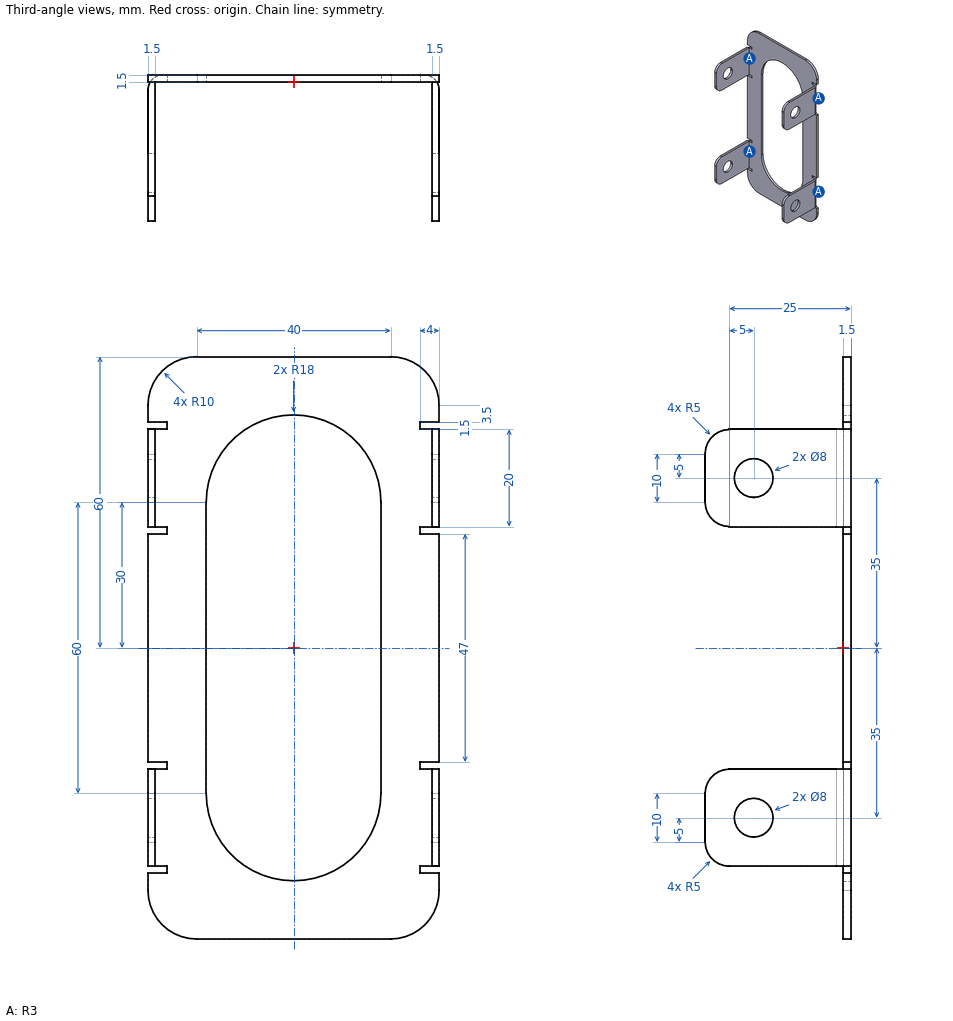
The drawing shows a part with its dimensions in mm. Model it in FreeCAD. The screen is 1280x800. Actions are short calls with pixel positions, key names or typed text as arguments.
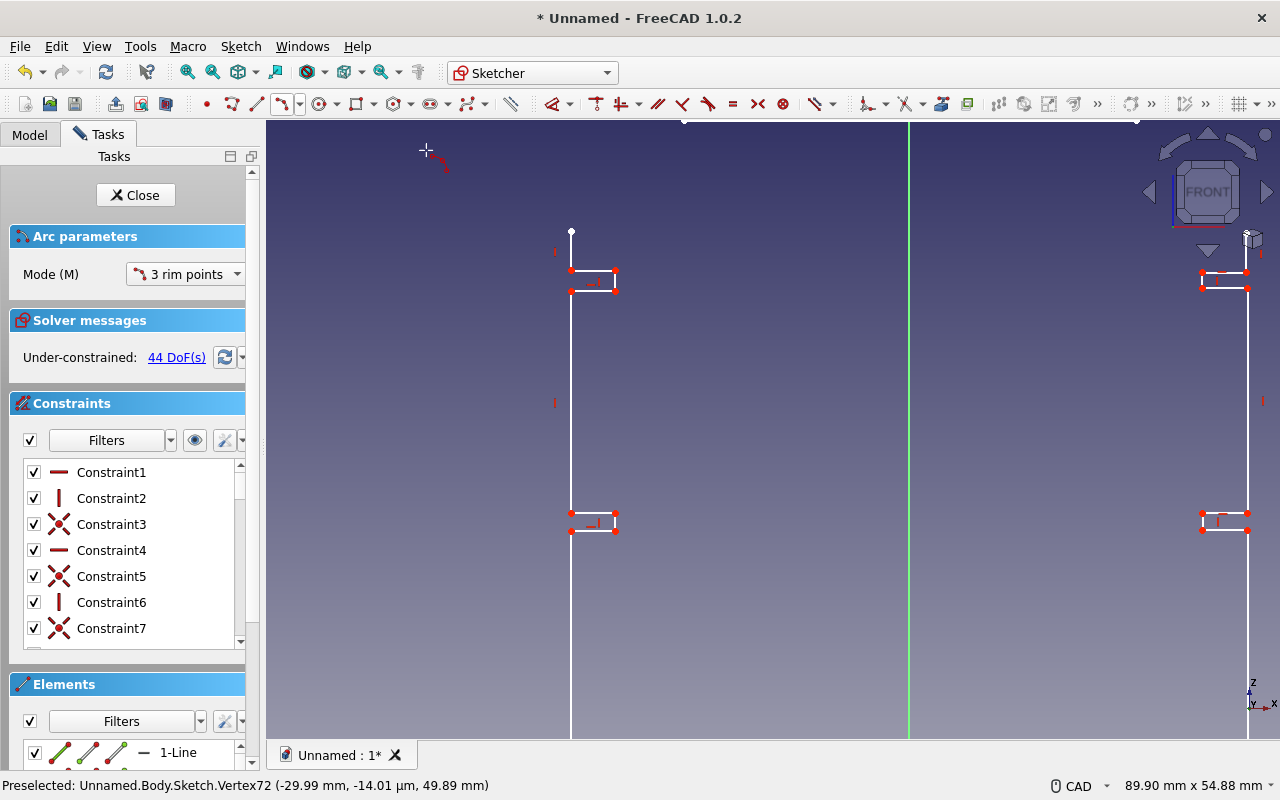
scroll(616, 272, down, 6)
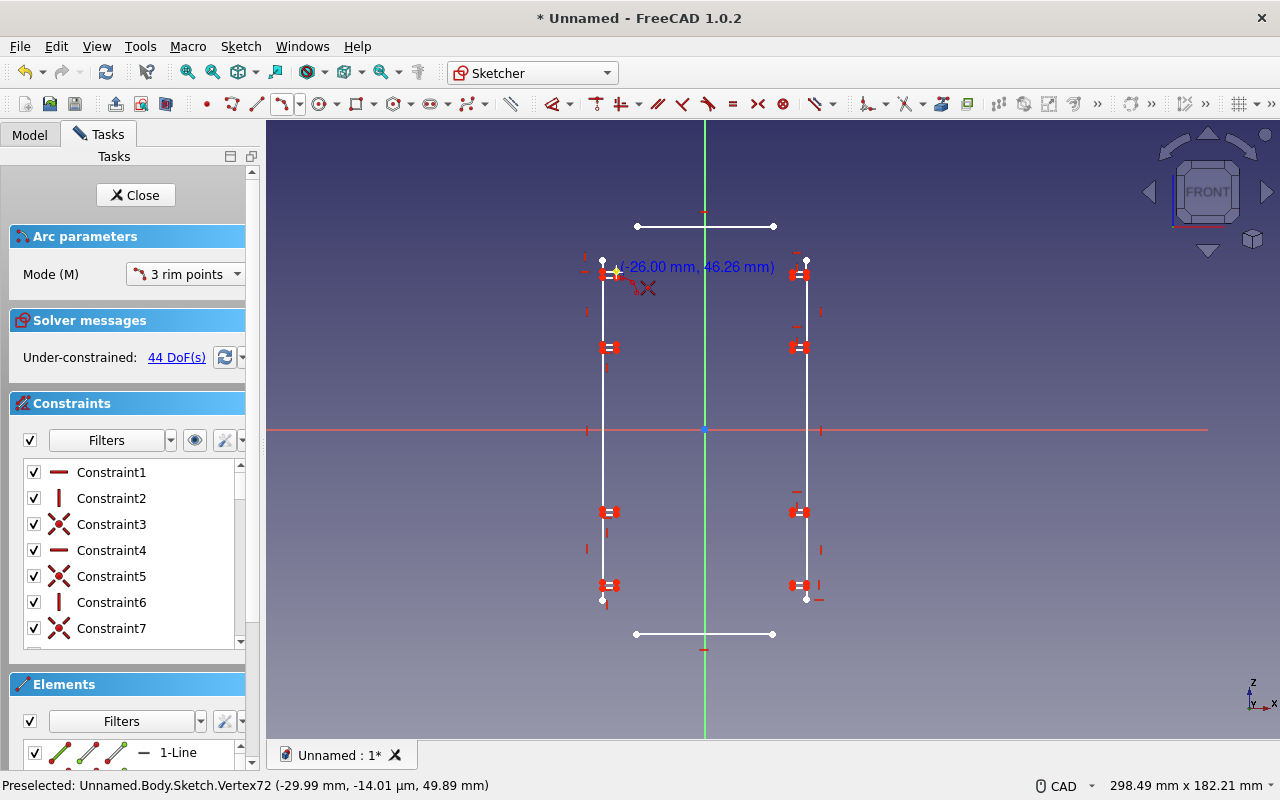
click(773, 227)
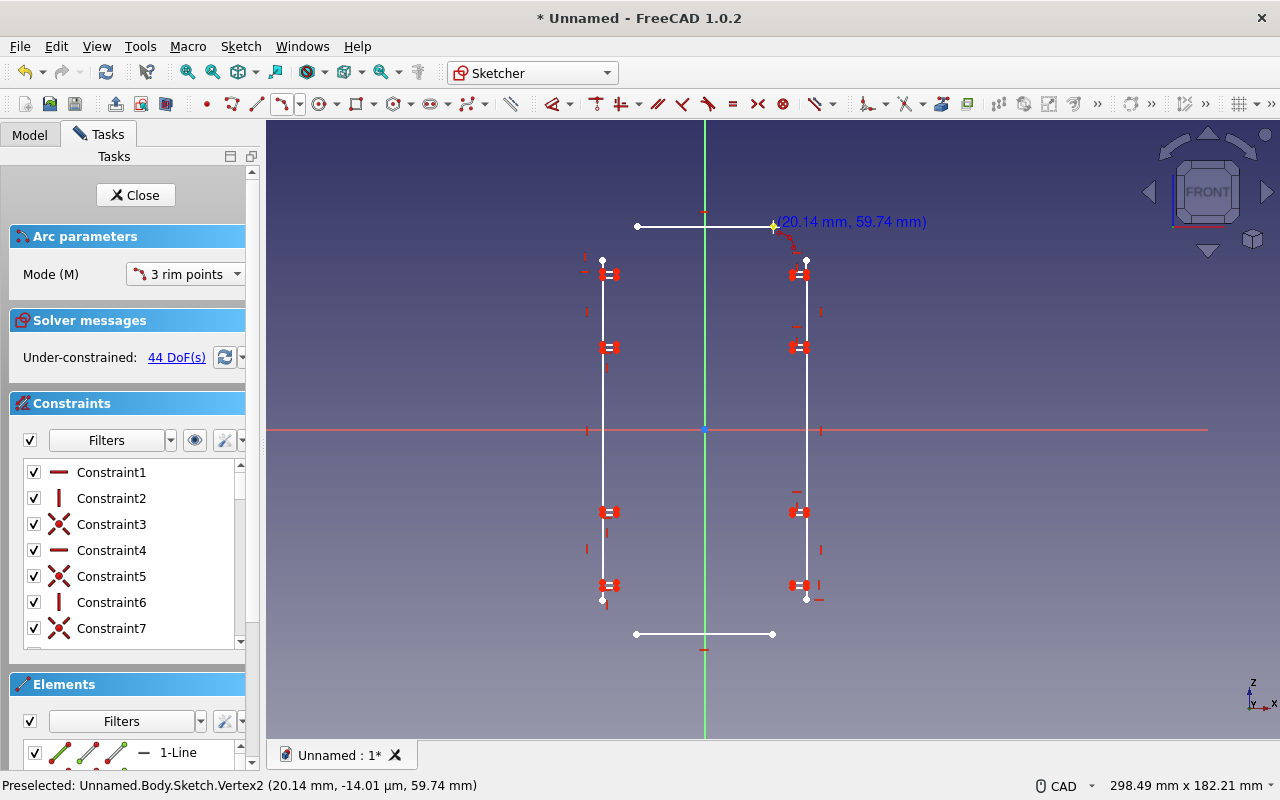
scroll(806, 260, up, 5)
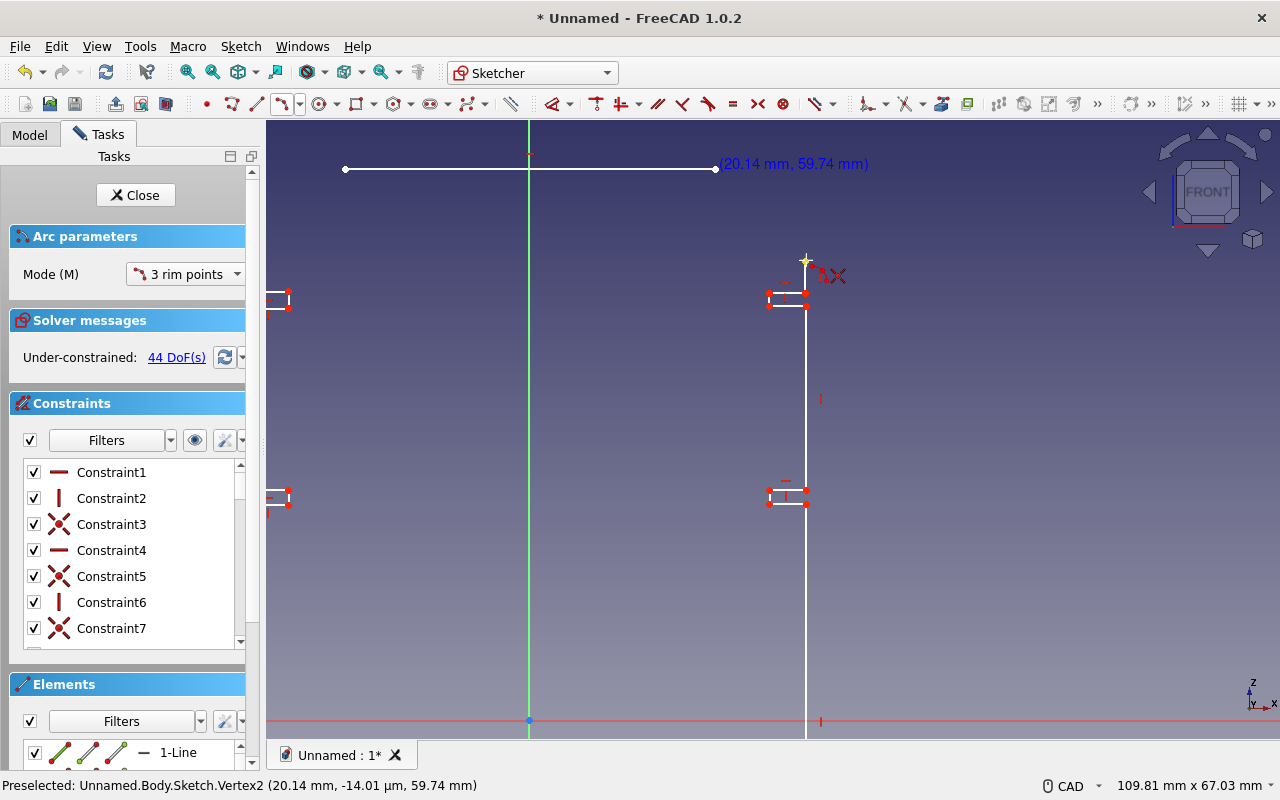
click(805, 261)
click(779, 194)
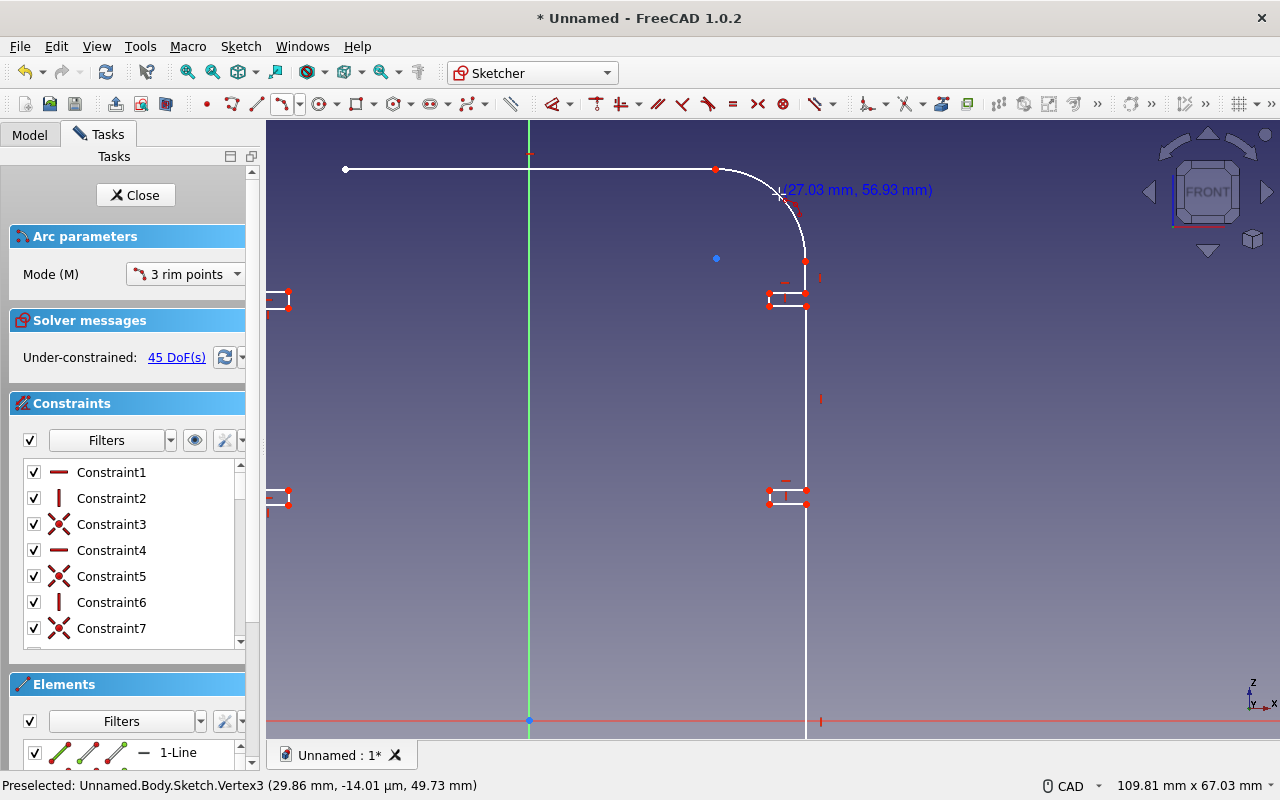
scroll(806, 260, down, 5)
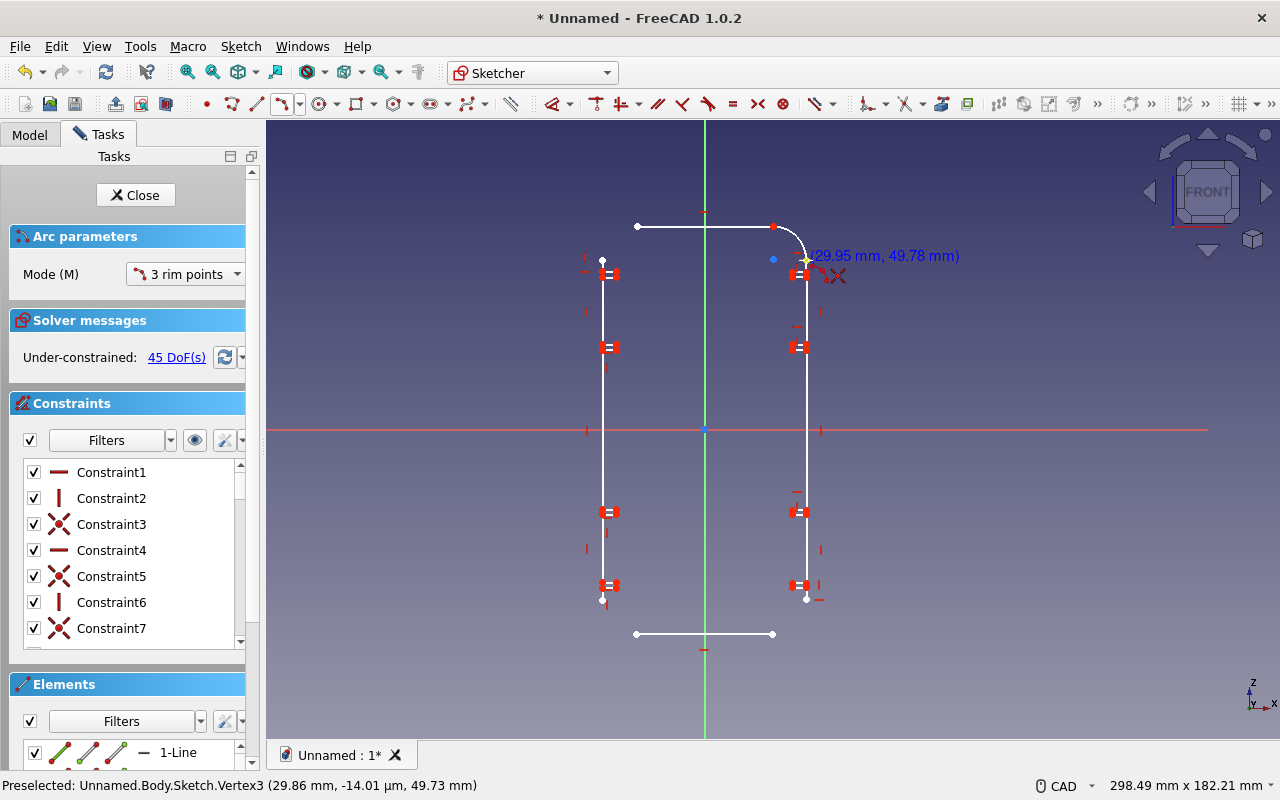
scroll(806, 599, up, 5)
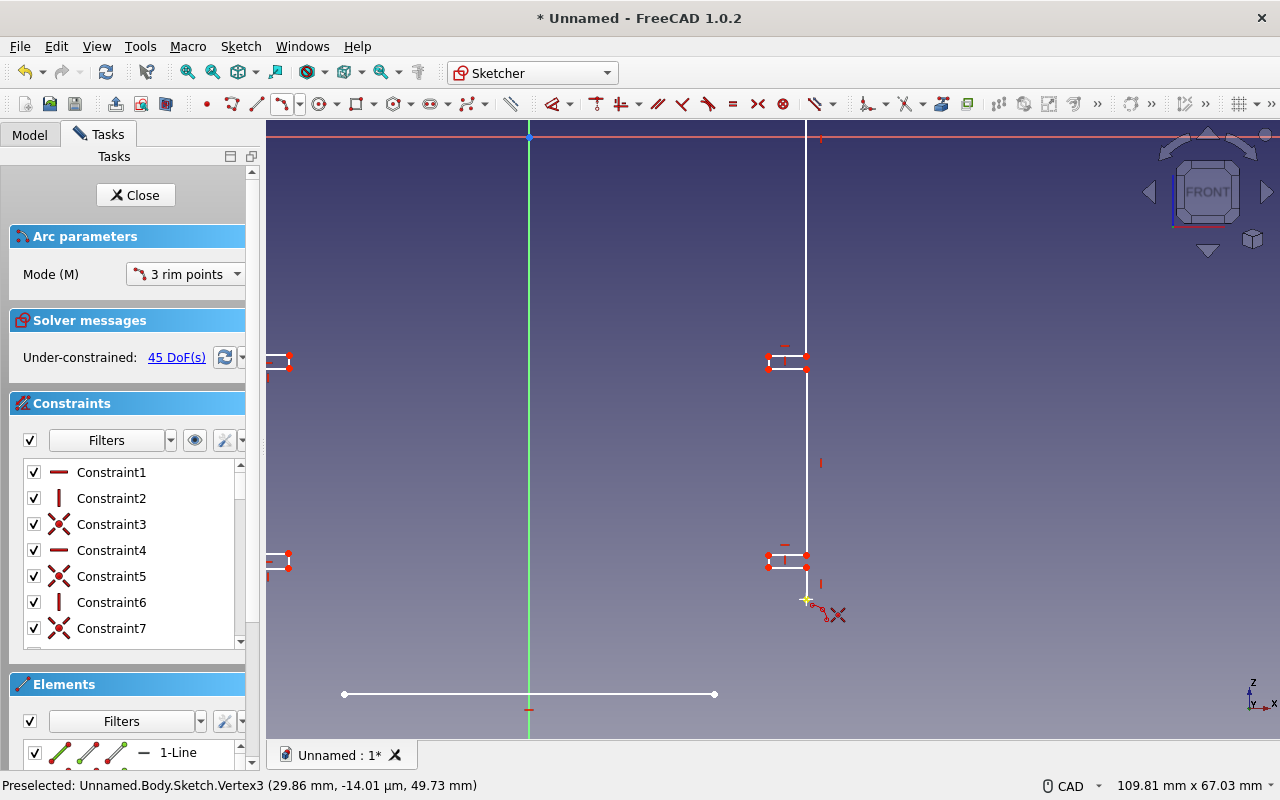
click(807, 600)
click(714, 694)
click(779, 664)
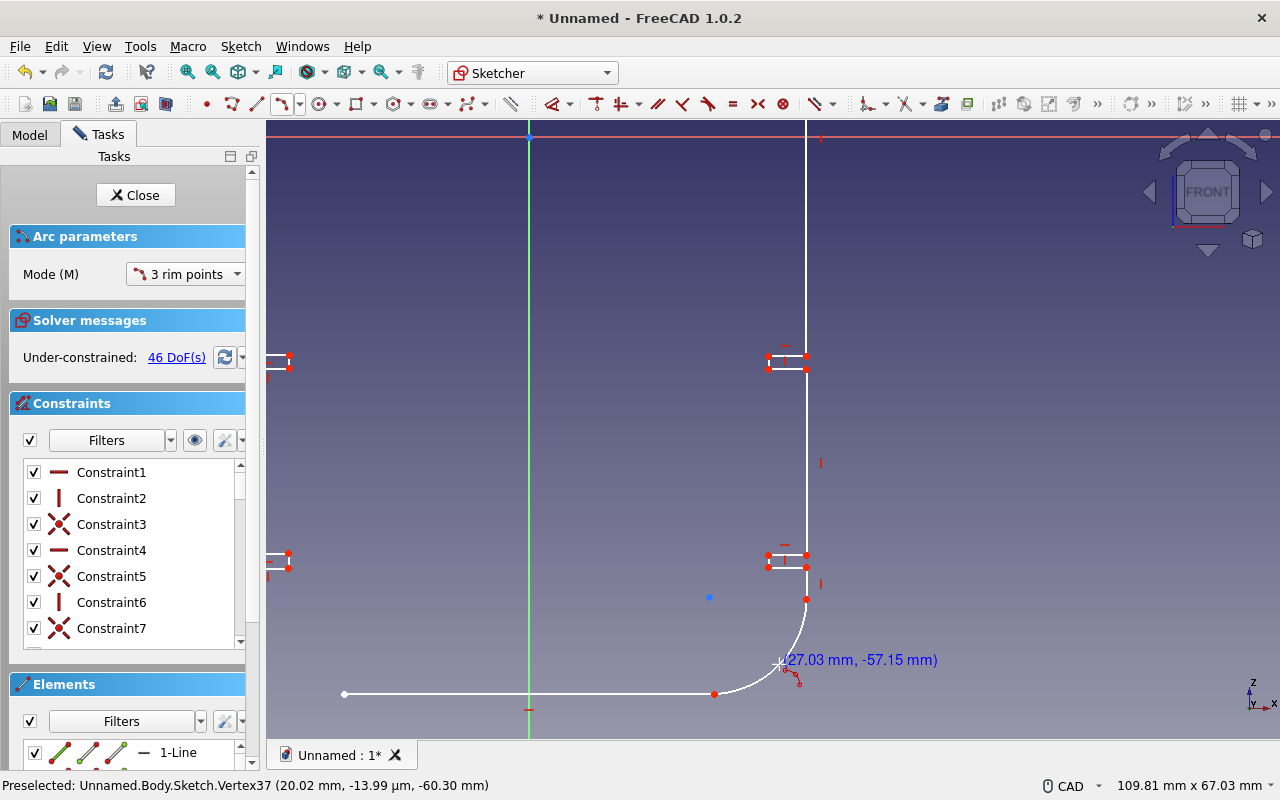
click(345, 694)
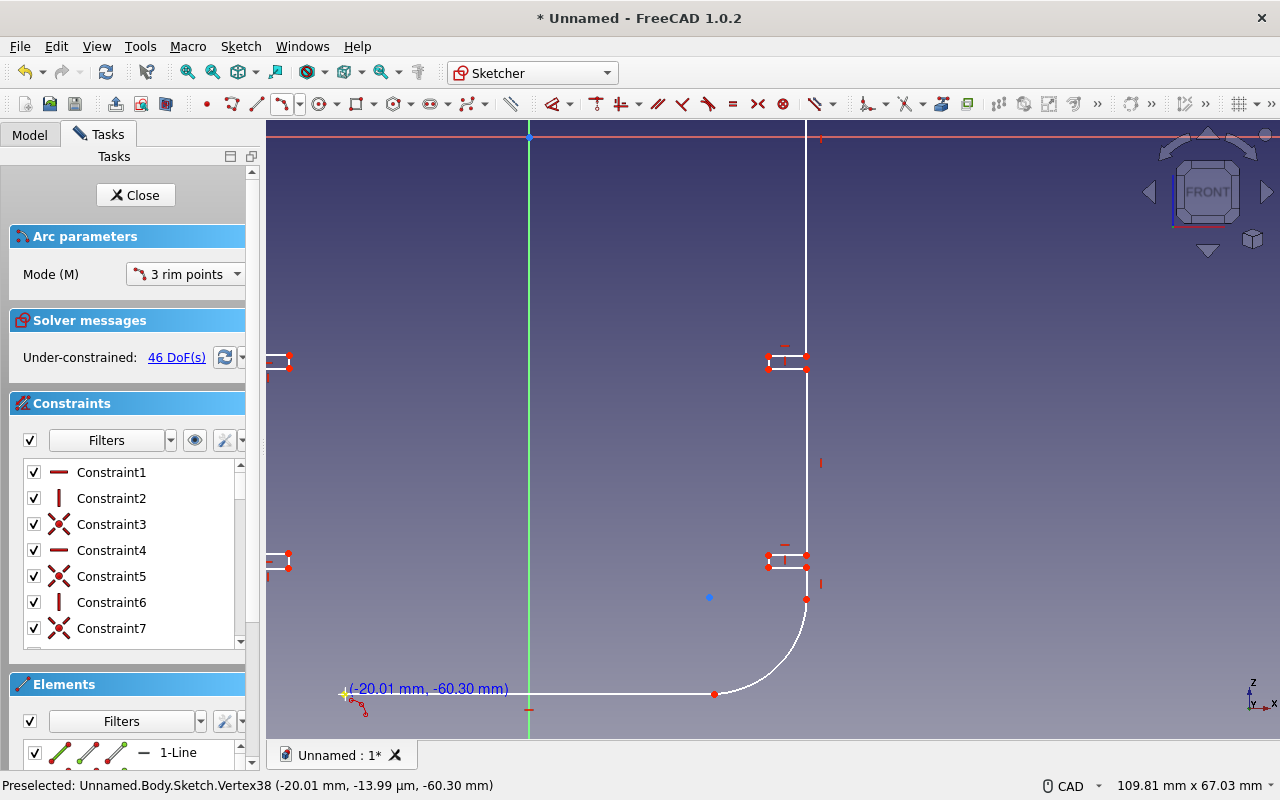
scroll(806, 600, down, 5)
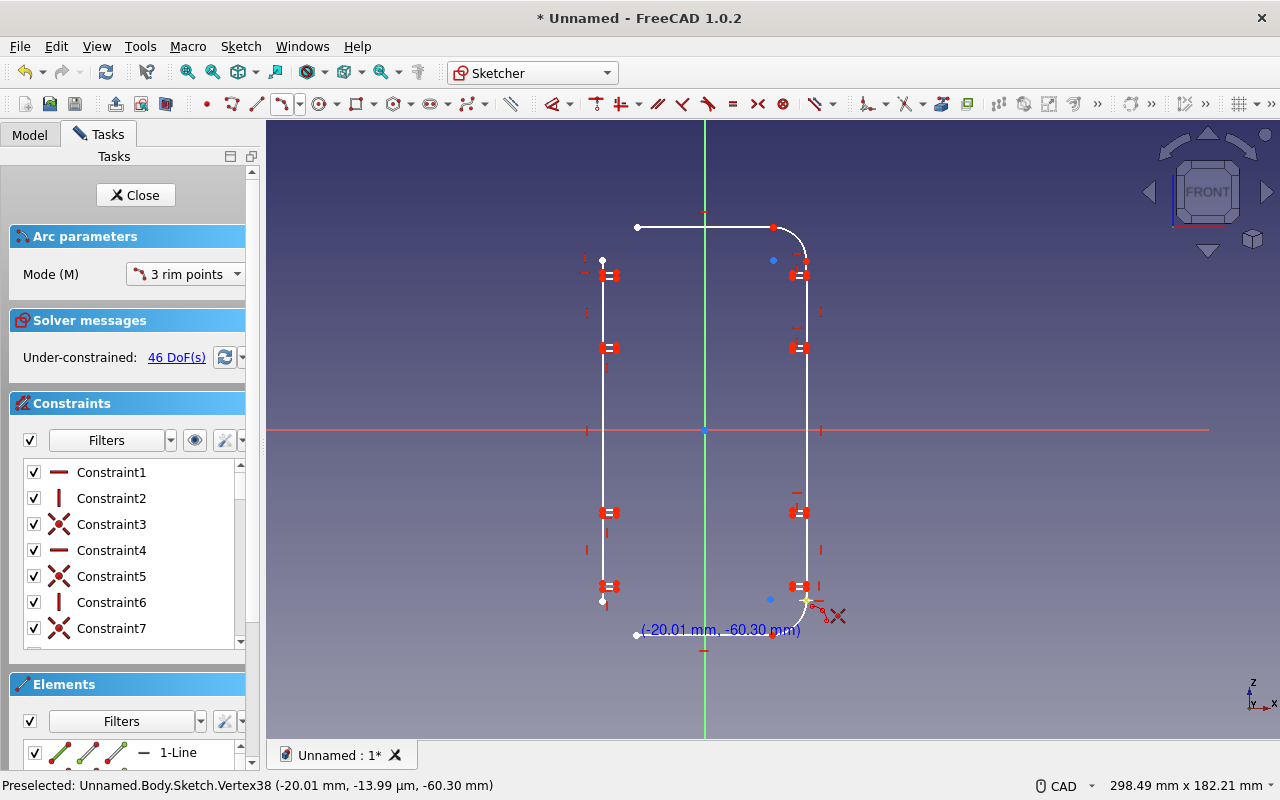
scroll(603, 600, up, 5)